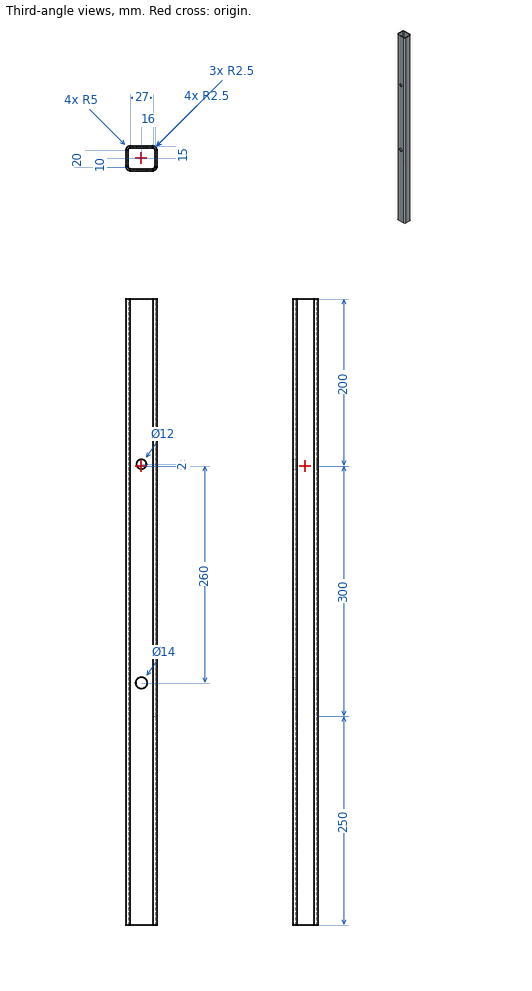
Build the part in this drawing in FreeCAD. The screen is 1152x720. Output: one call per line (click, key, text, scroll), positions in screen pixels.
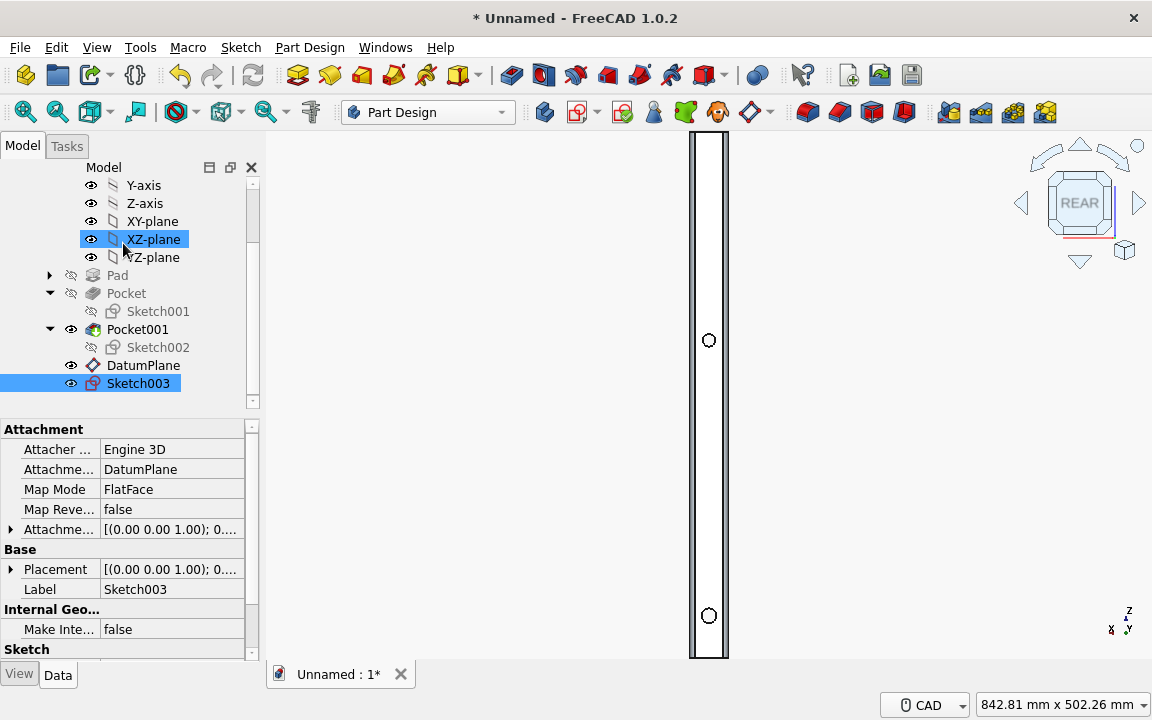
click(298, 76)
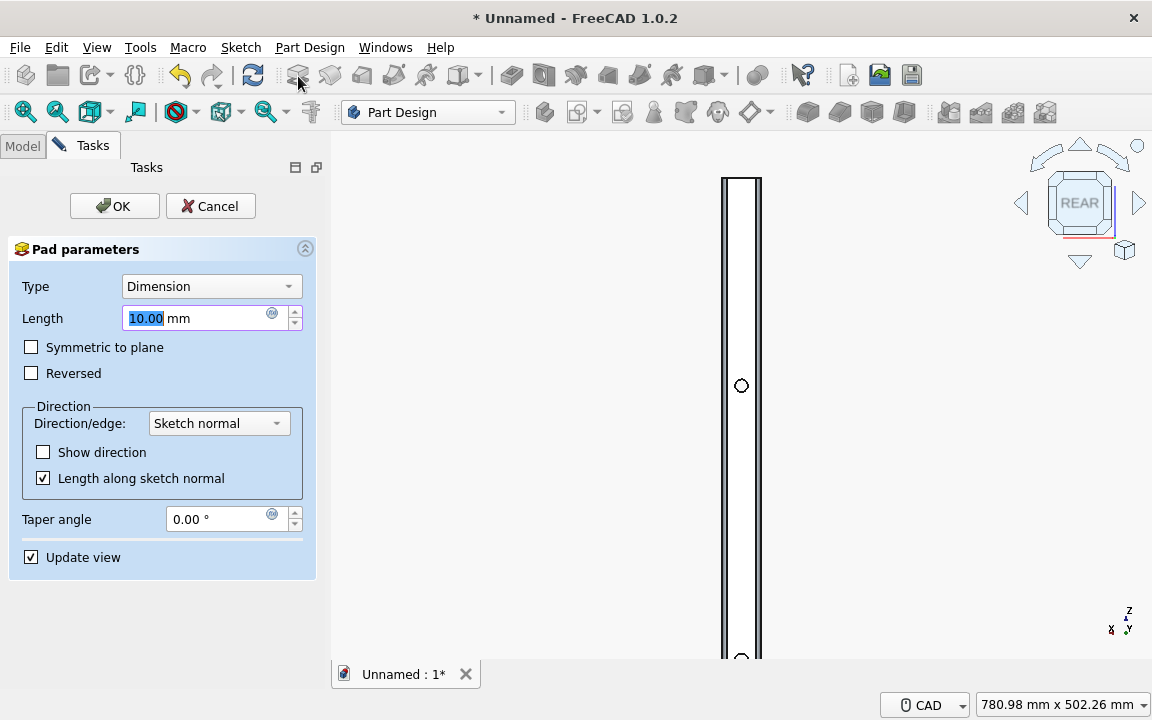
text(250)
key(Tab)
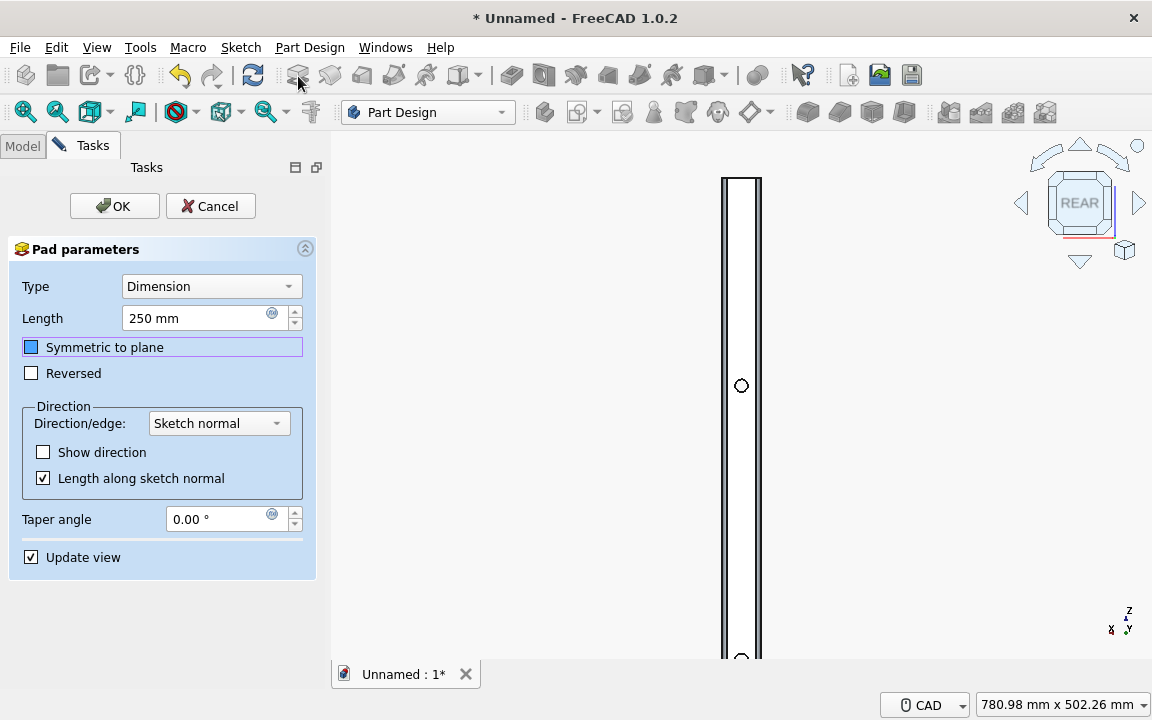
click(115, 206)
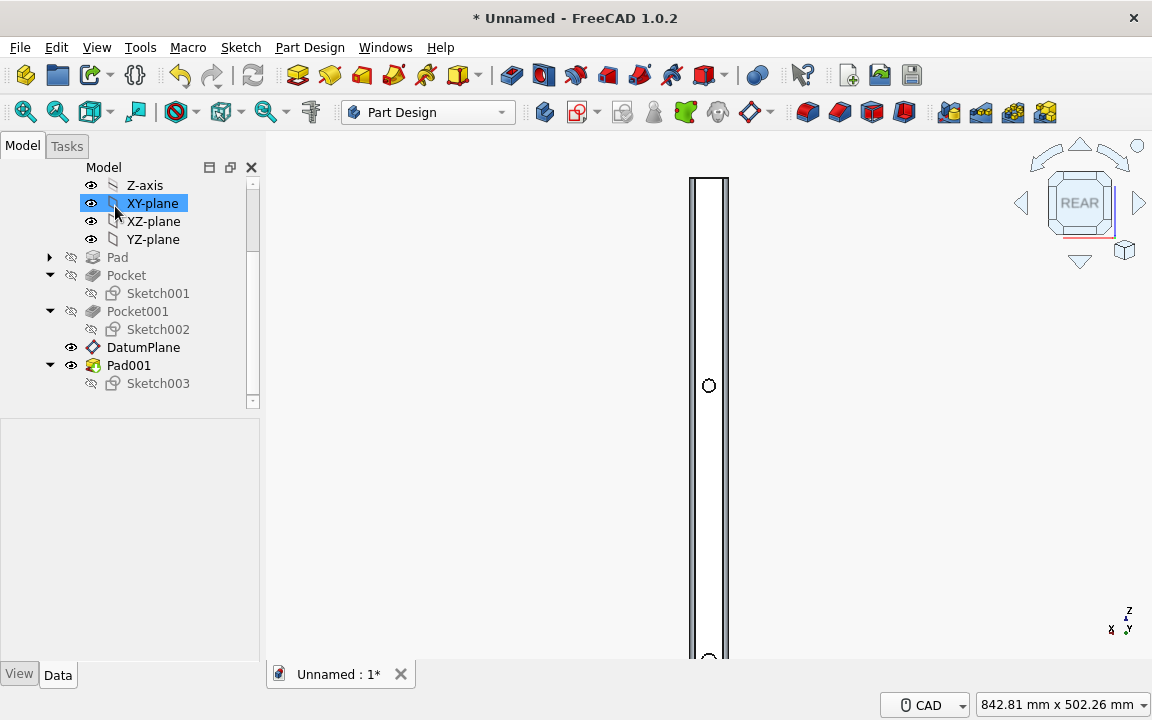
click(116, 347)
key(space)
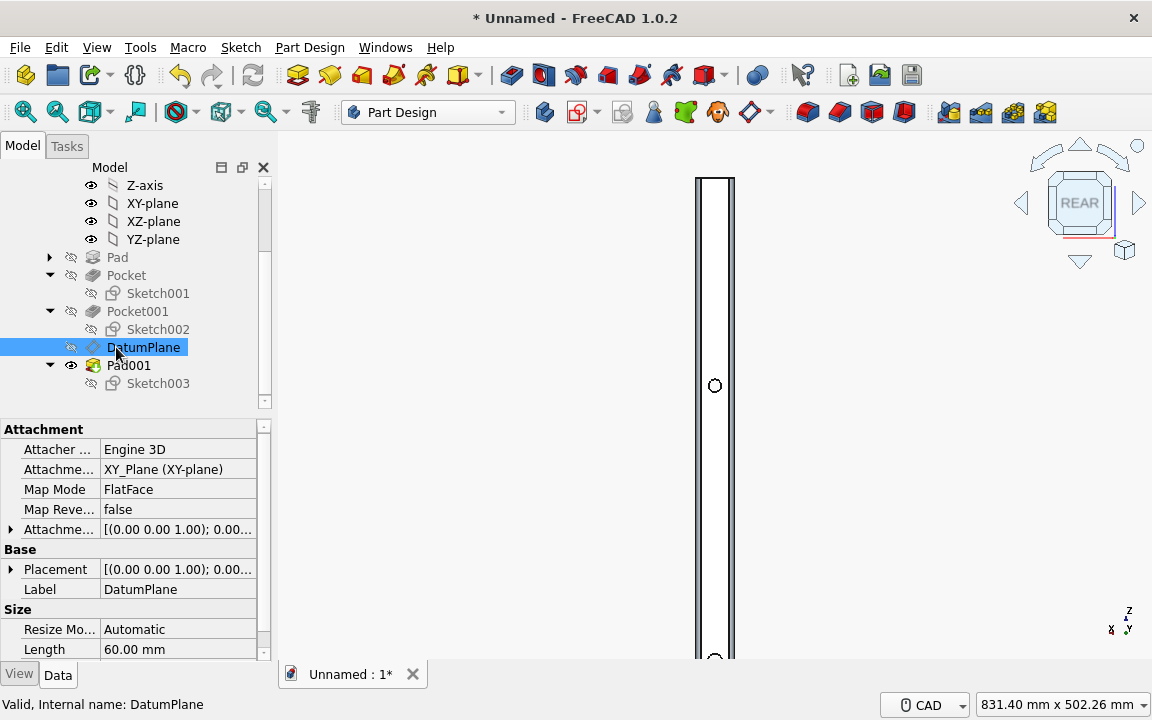
key(0)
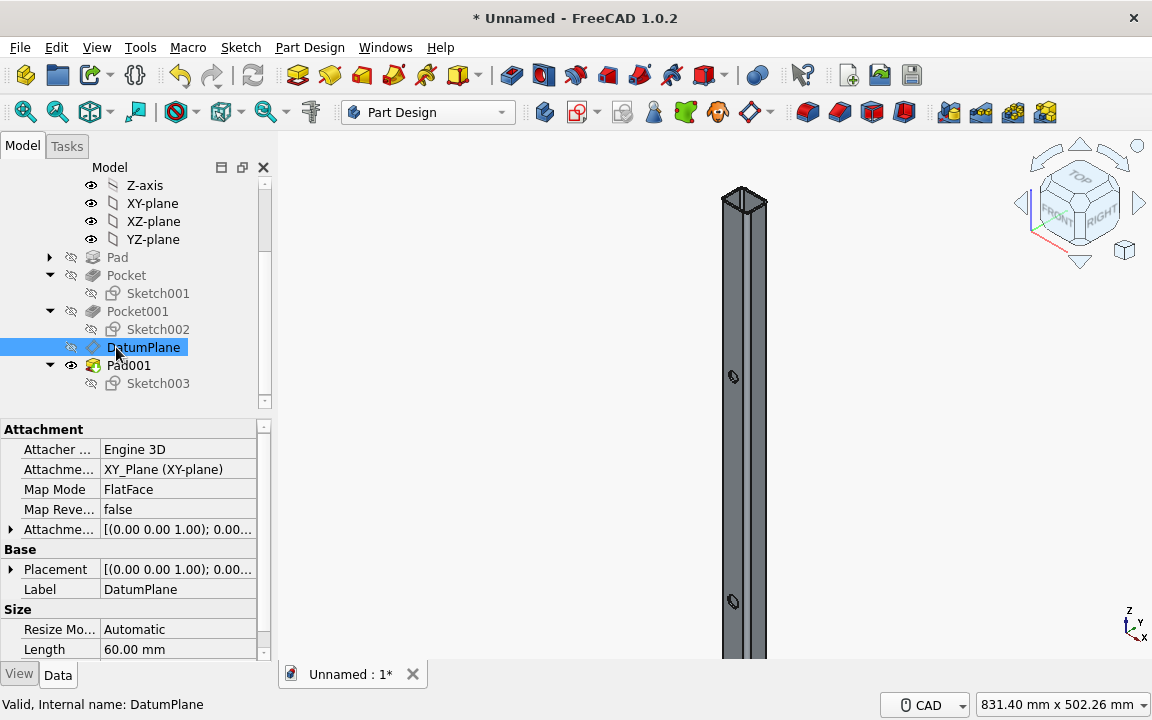
key(v)
key(f)